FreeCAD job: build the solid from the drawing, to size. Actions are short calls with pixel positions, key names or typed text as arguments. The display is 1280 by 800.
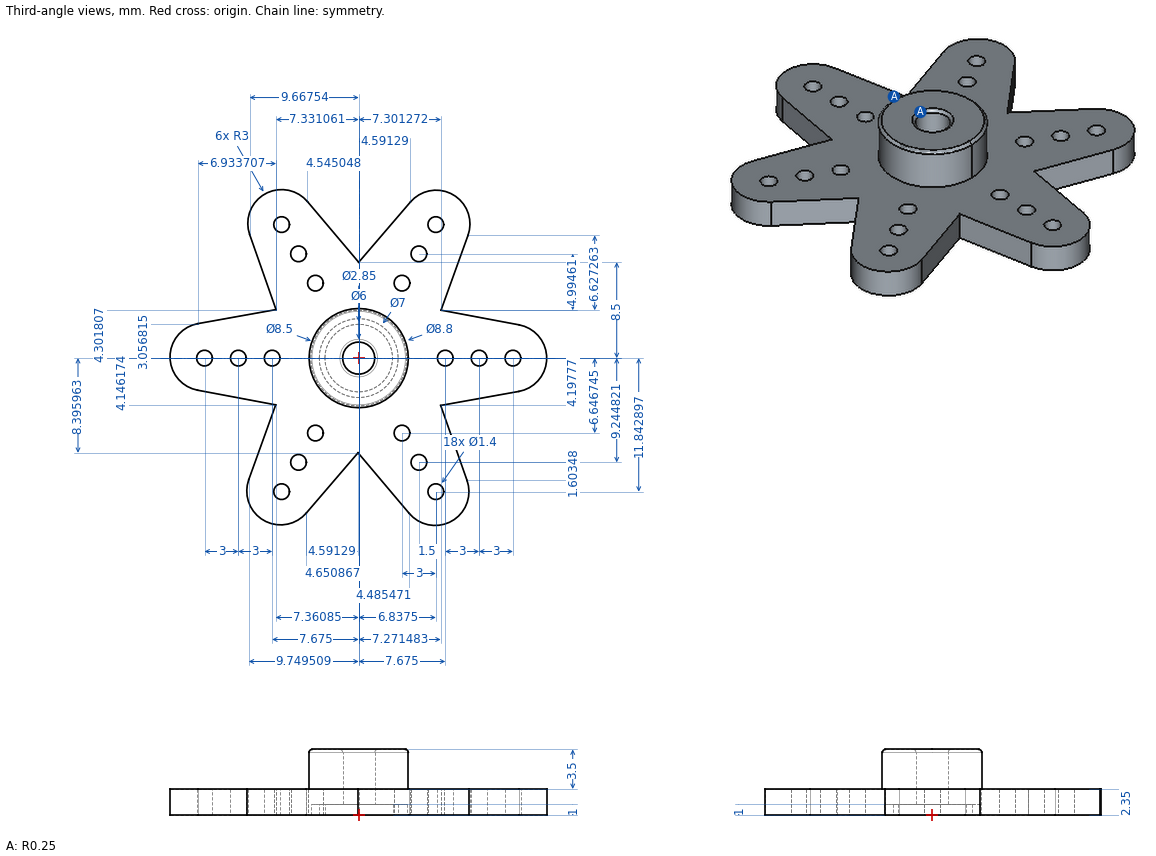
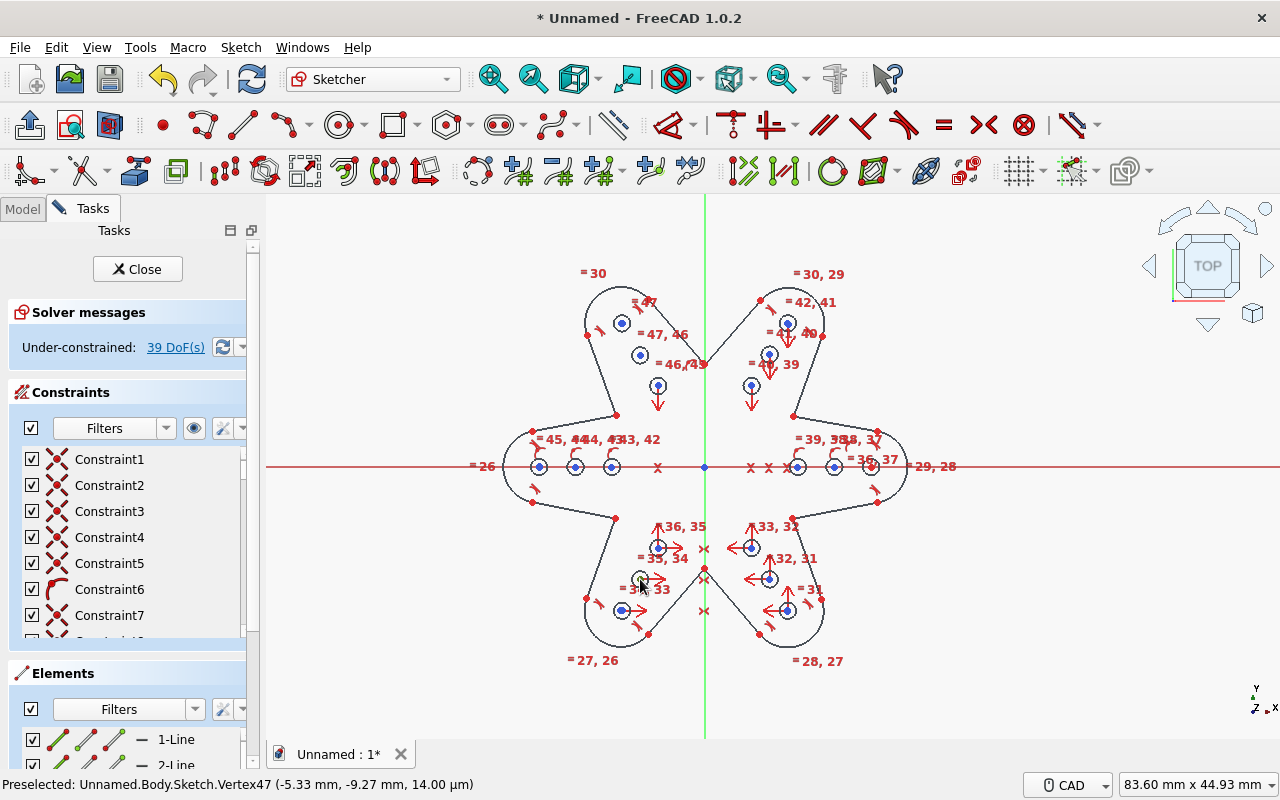
click(640, 355)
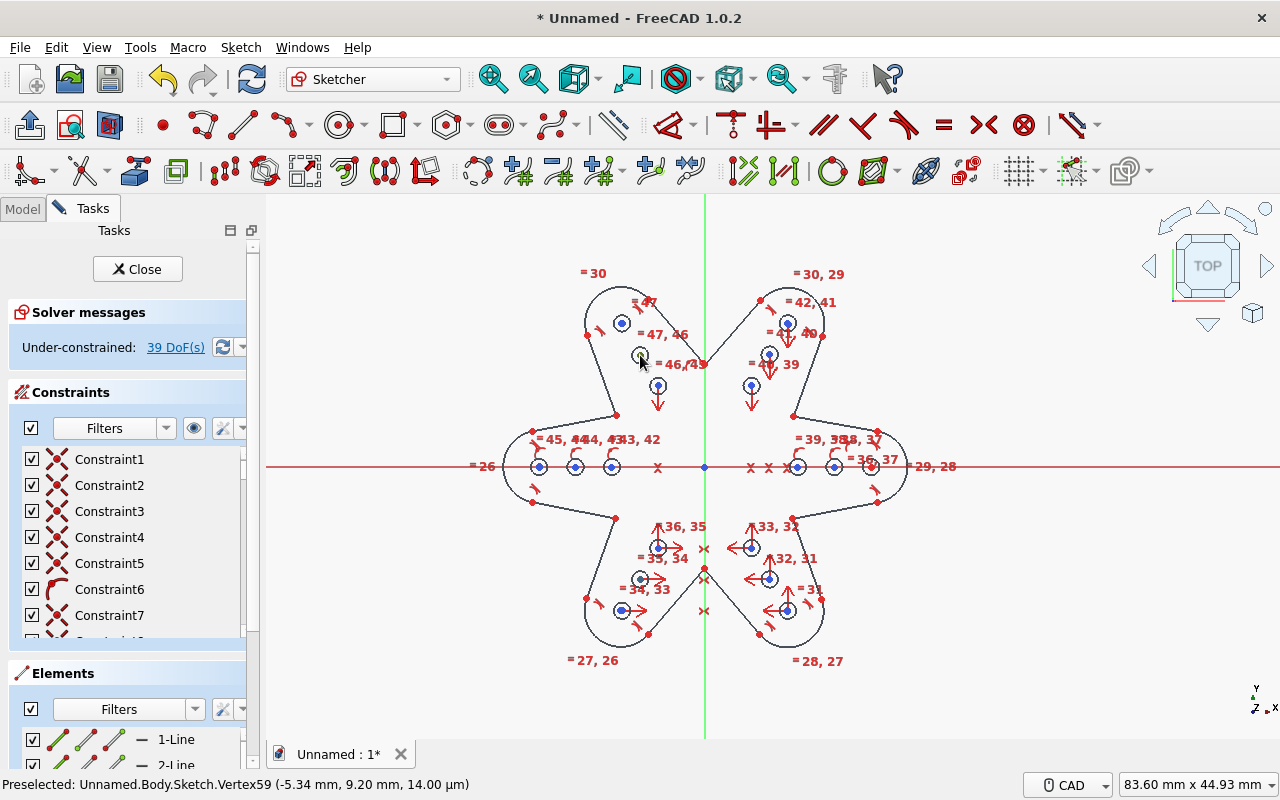
click(353, 467)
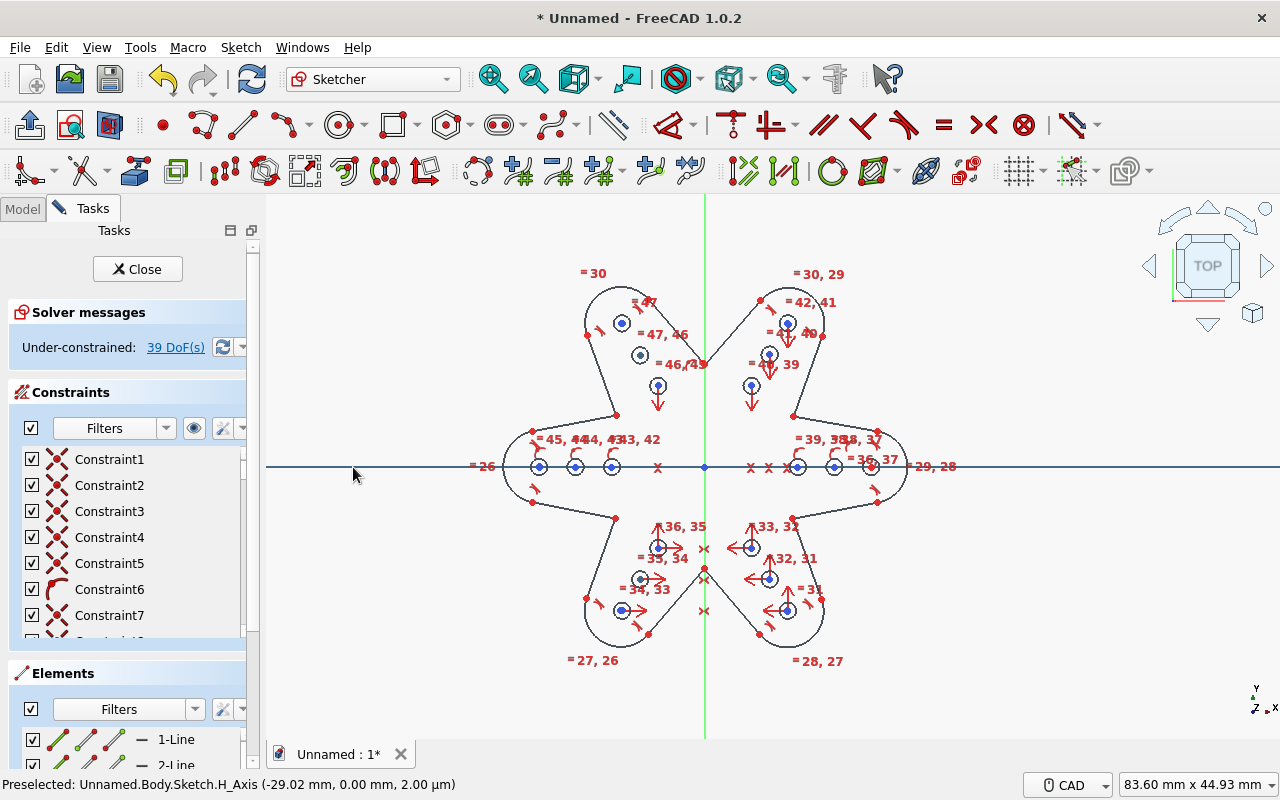
click(984, 126)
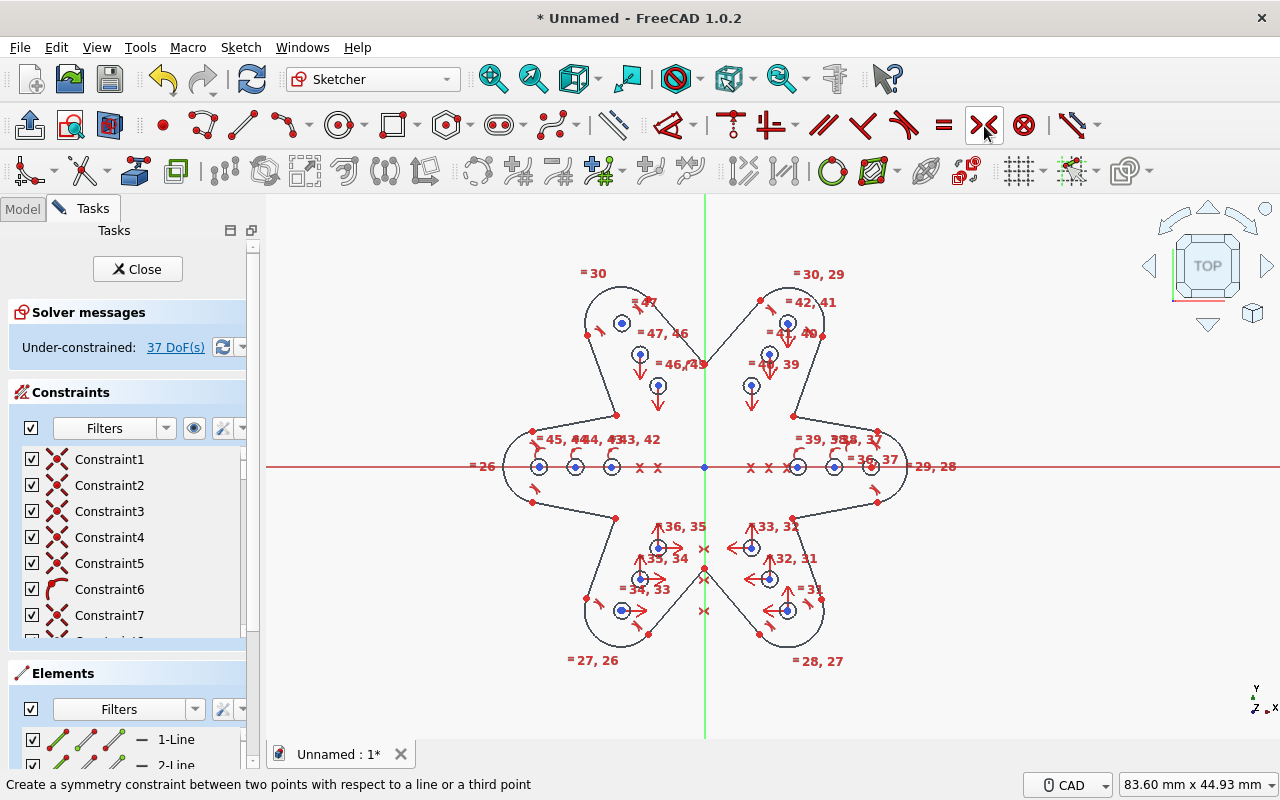
scroll(622, 611, up, 12)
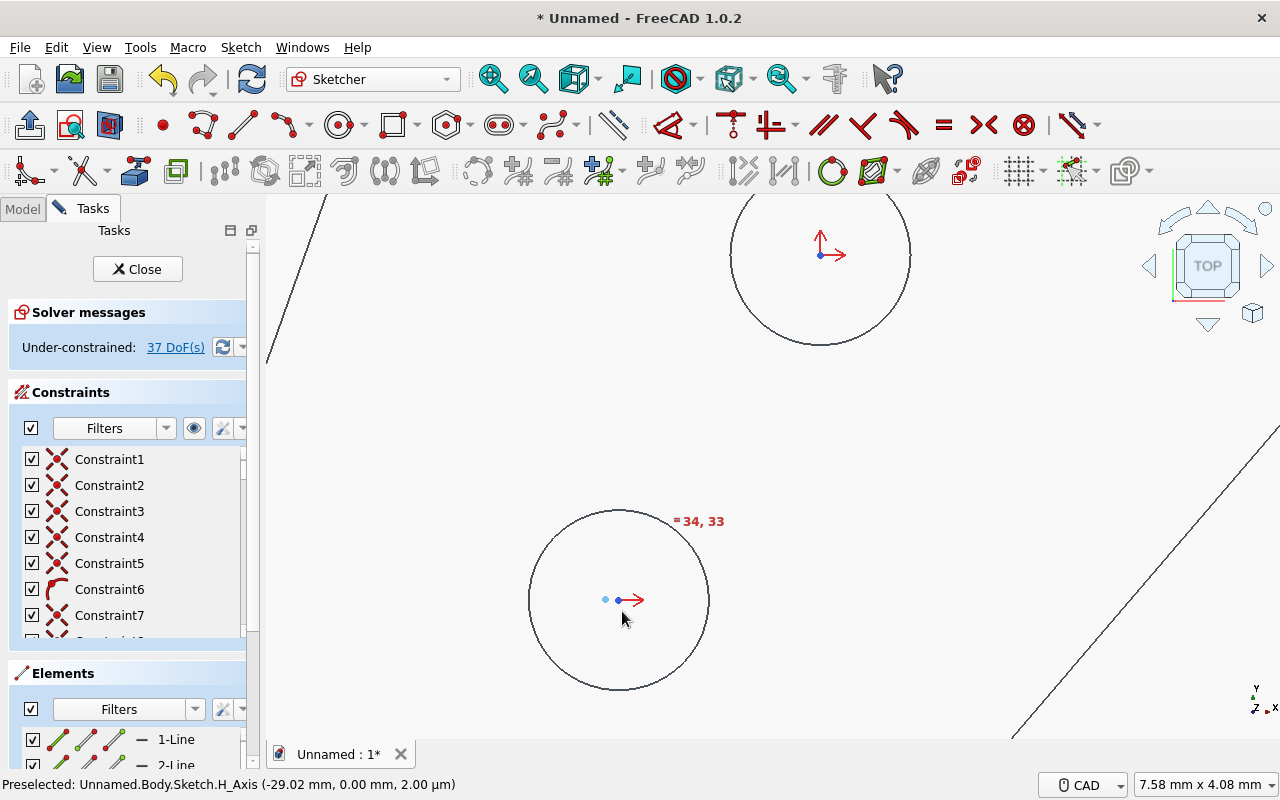
click(619, 600)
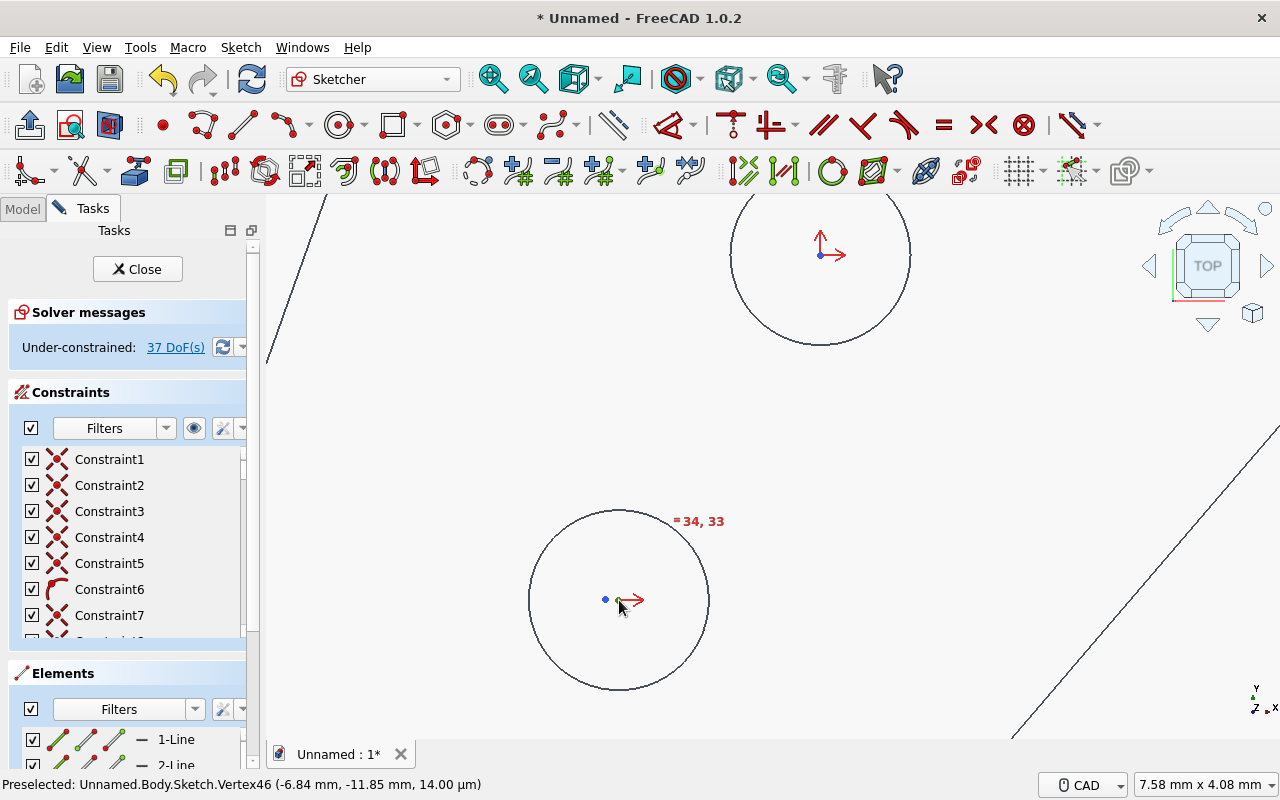
scroll(622, 612, down, 12)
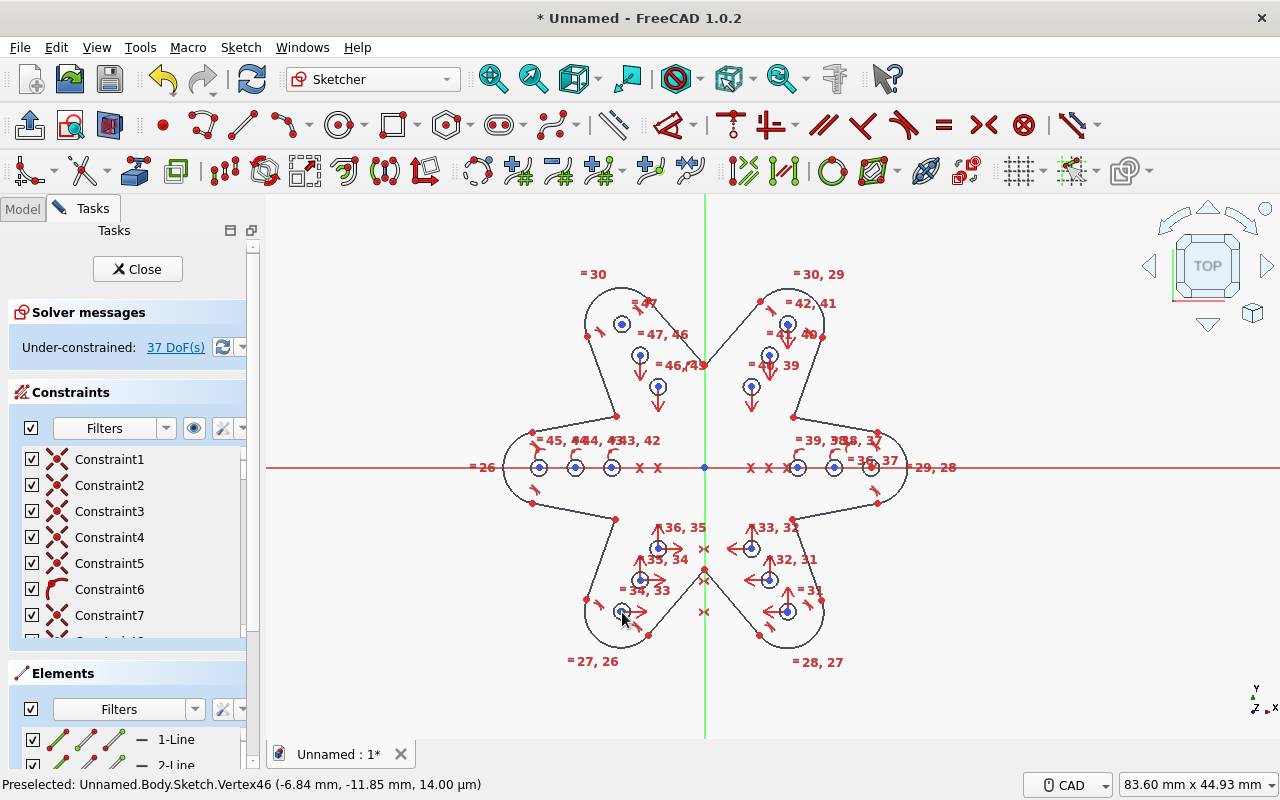
scroll(622, 324, up, 14)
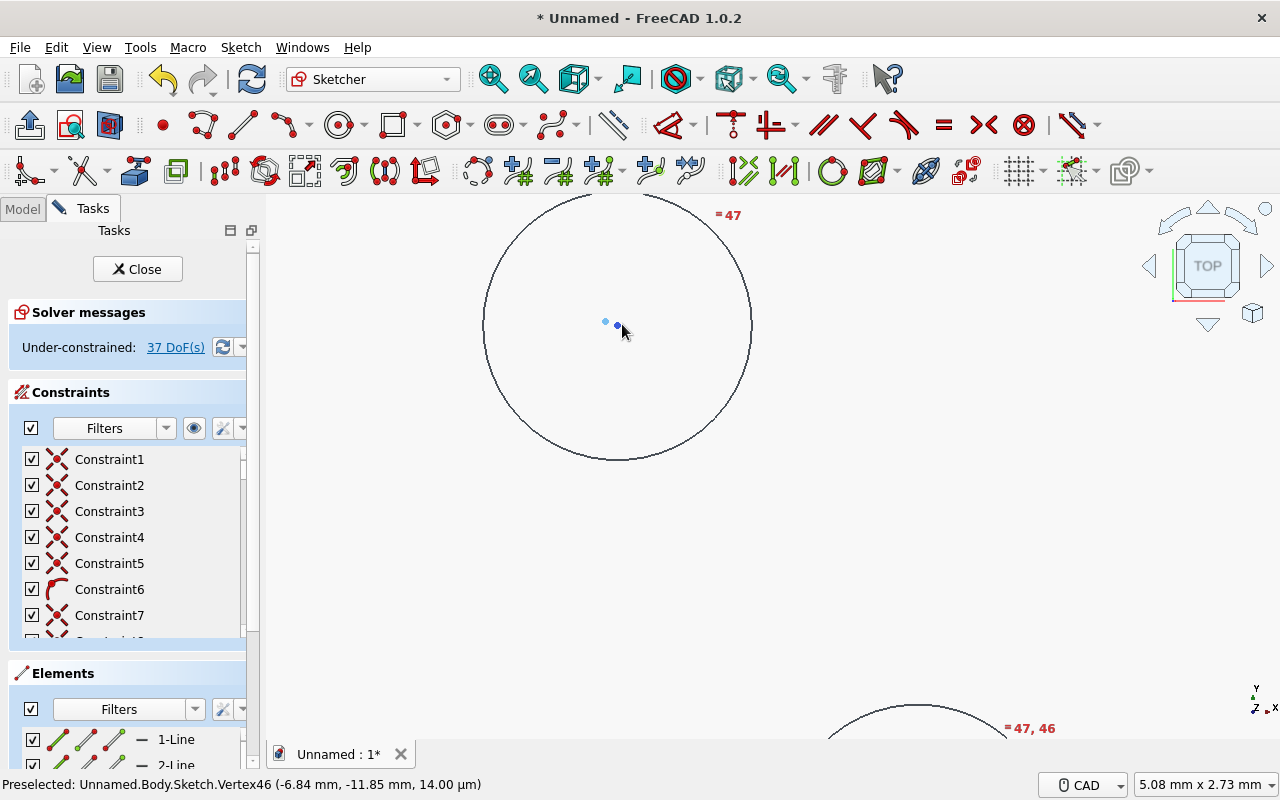
click(617, 326)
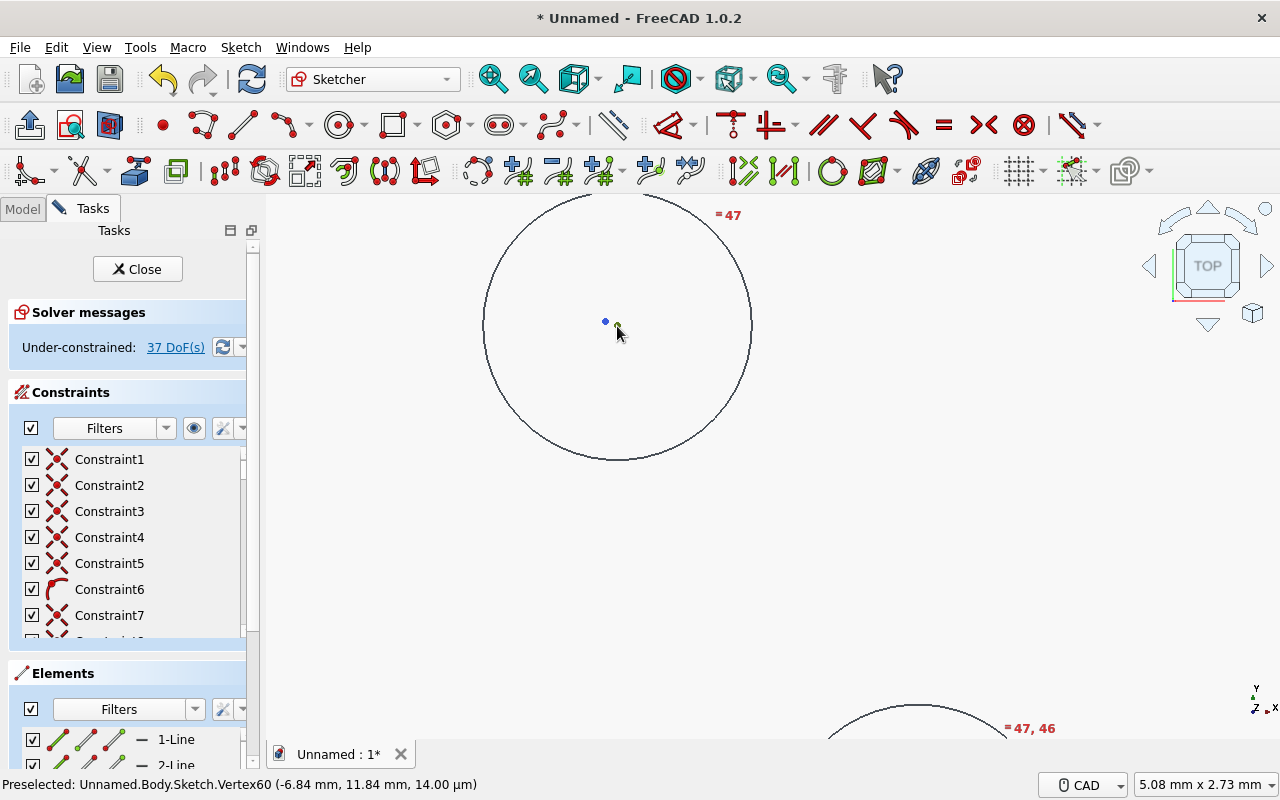
scroll(622, 323, down, 14)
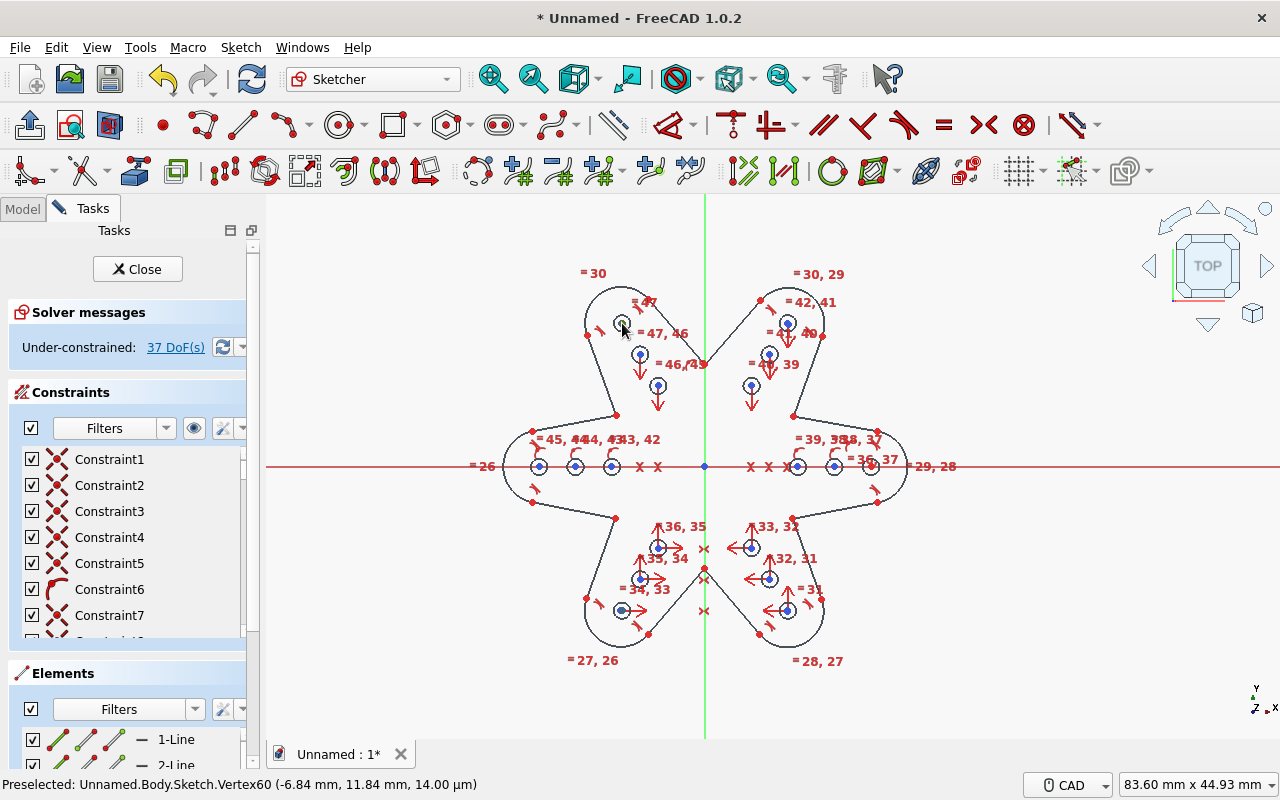
click(353, 467)